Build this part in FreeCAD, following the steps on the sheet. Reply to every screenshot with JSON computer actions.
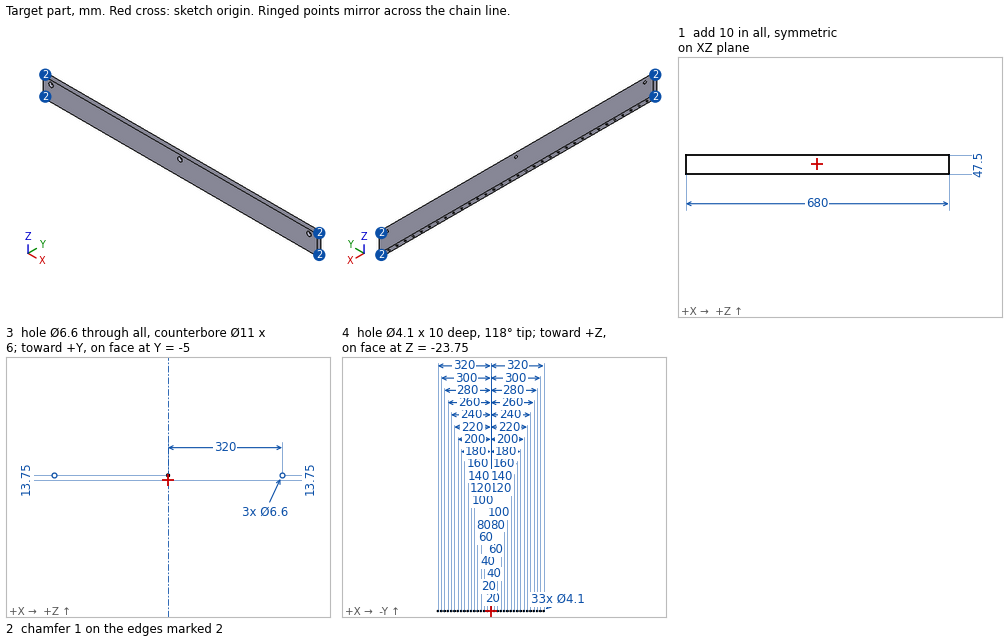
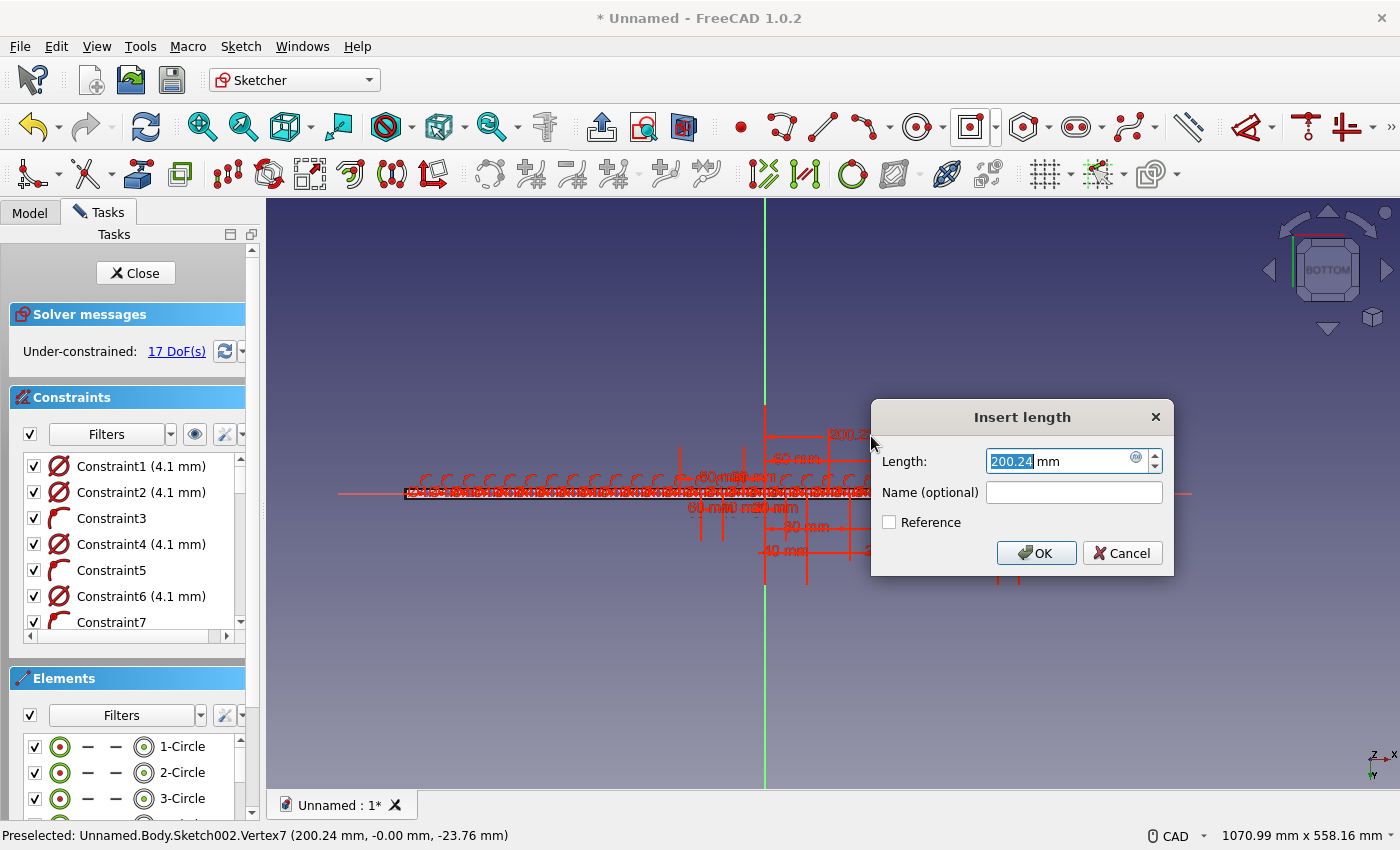
{"action": "type", "text": "200"}
{"action": "key", "text": "Return"}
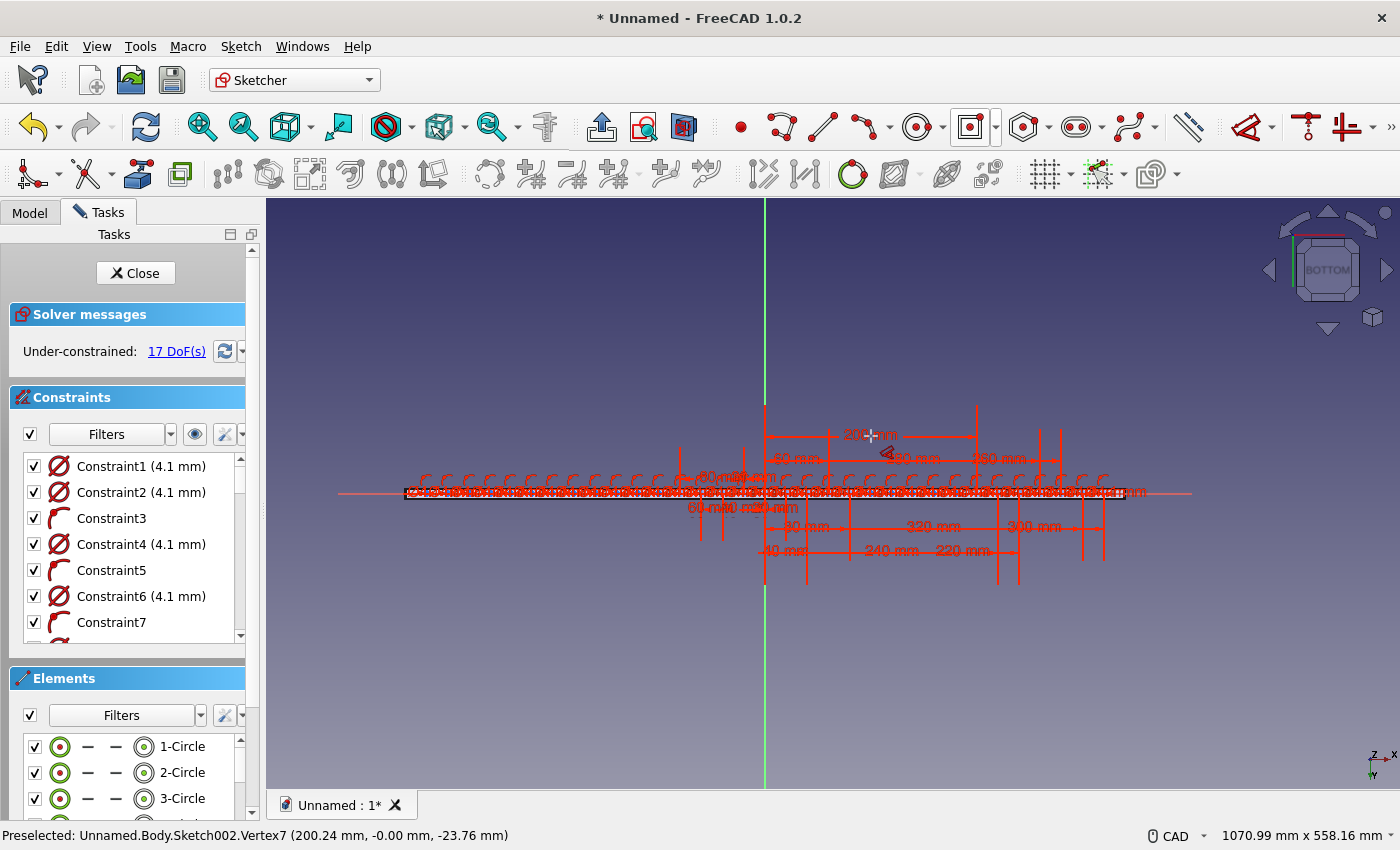
{"action": "left_click", "coordinate": [956, 494]}
{"action": "left_click", "coordinate": [794, 436]}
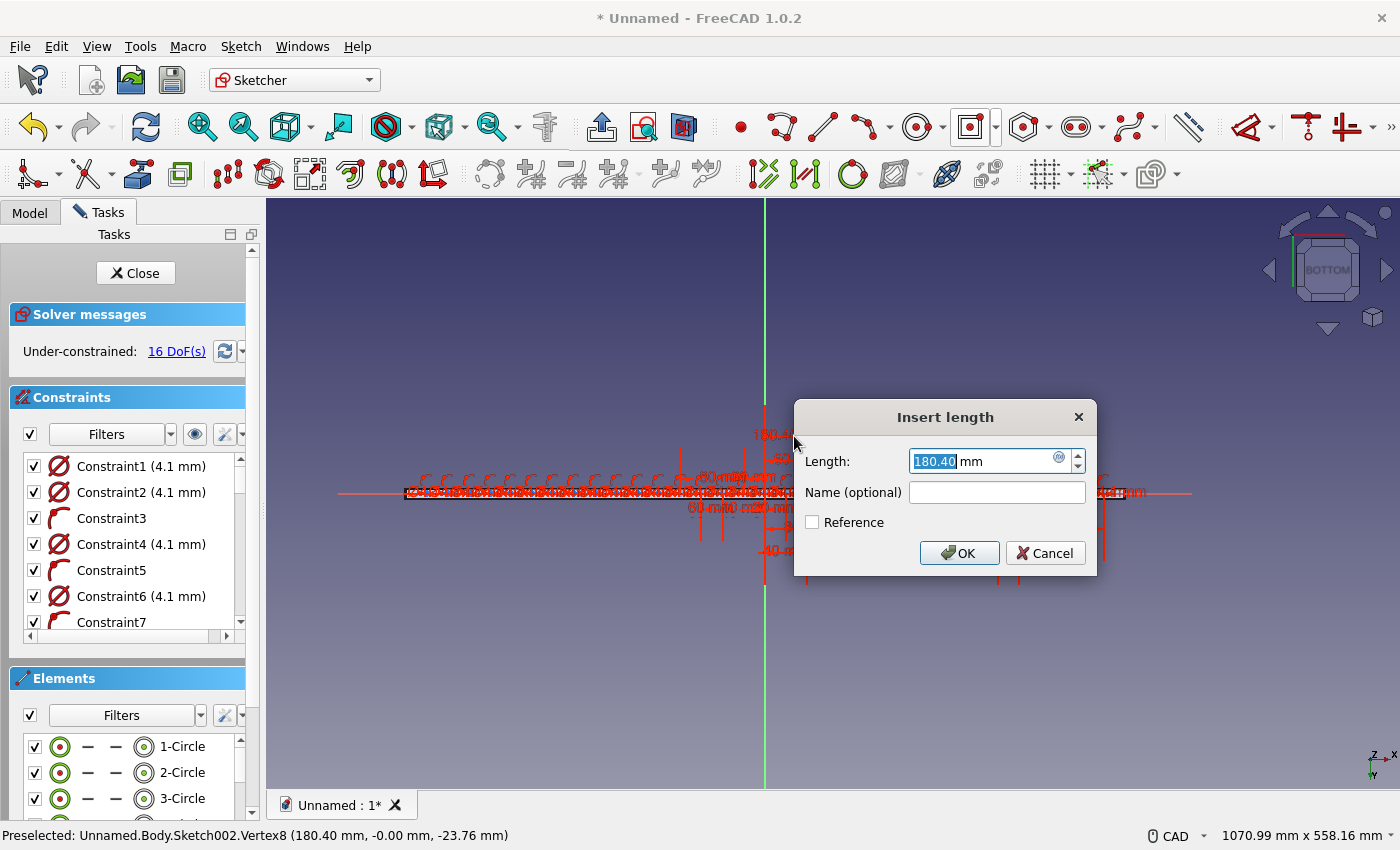
{"action": "type", "text": "180"}
{"action": "key", "text": "Return"}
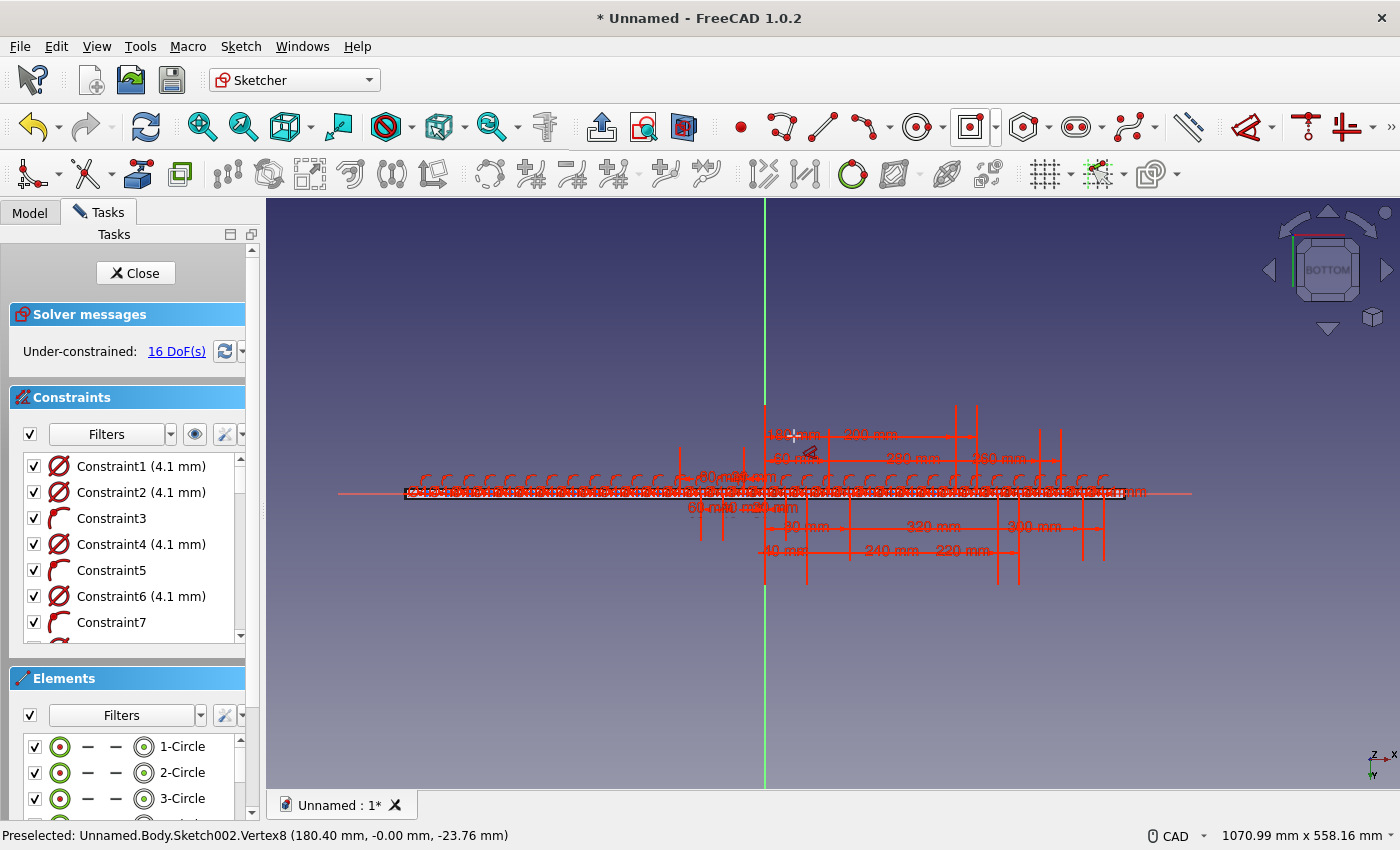
{"action": "left_click", "coordinate": [934, 494]}
{"action": "left_click", "coordinate": [849, 576]}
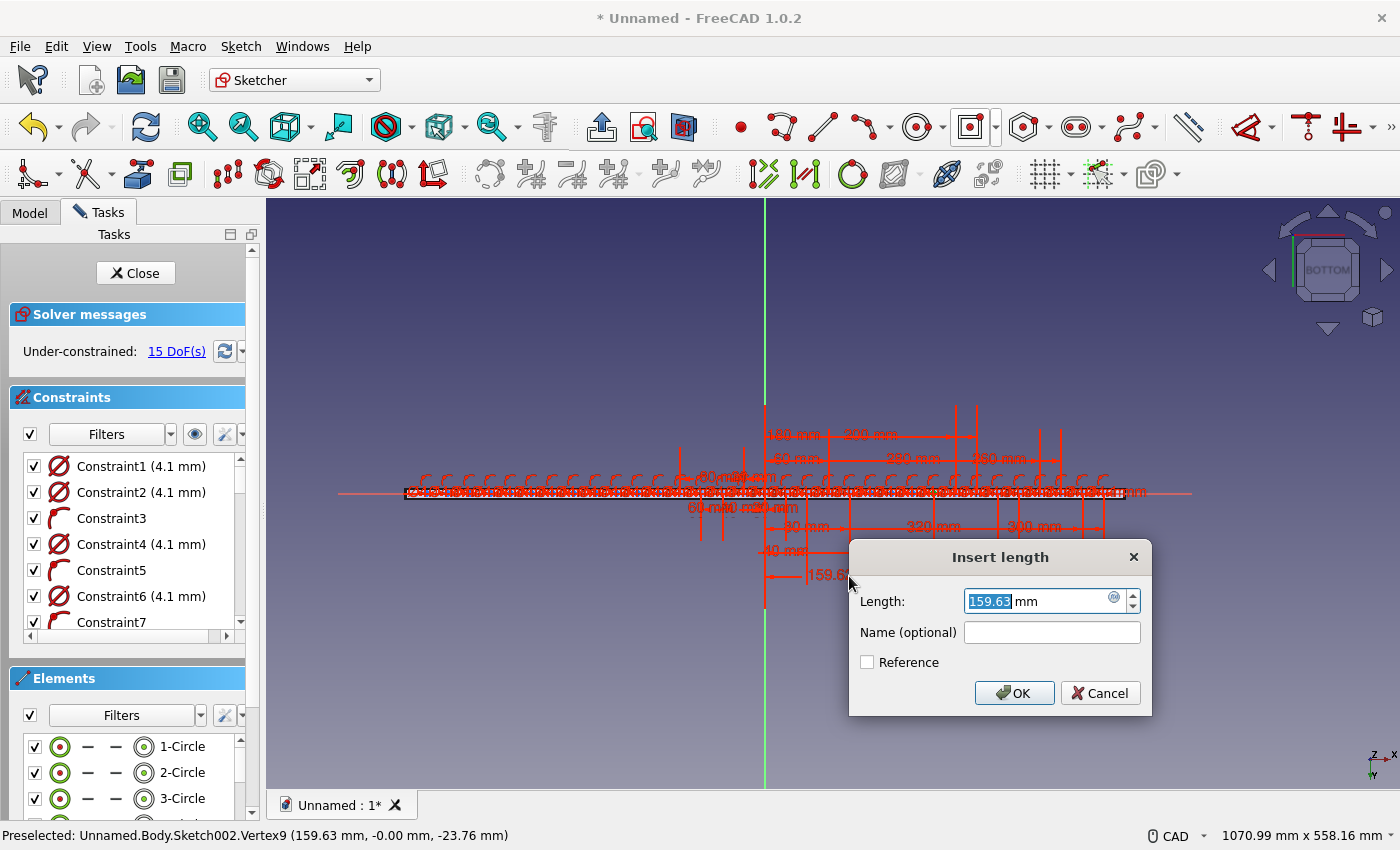
{"action": "type", "text": "160"}
{"action": "key", "text": "Return"}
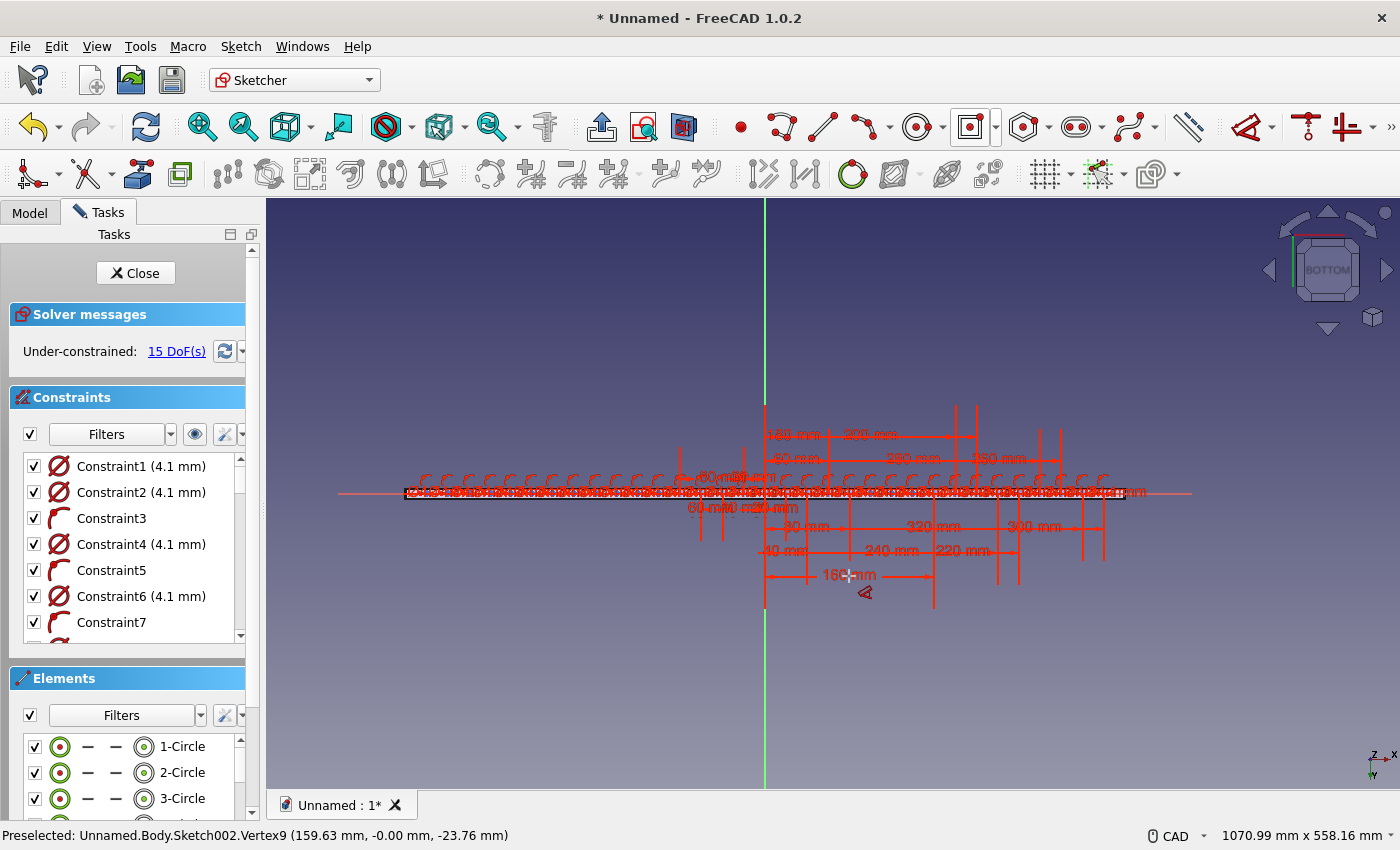
{"action": "left_click", "coordinate": [913, 494]}
{"action": "left_click", "coordinate": [839, 412]}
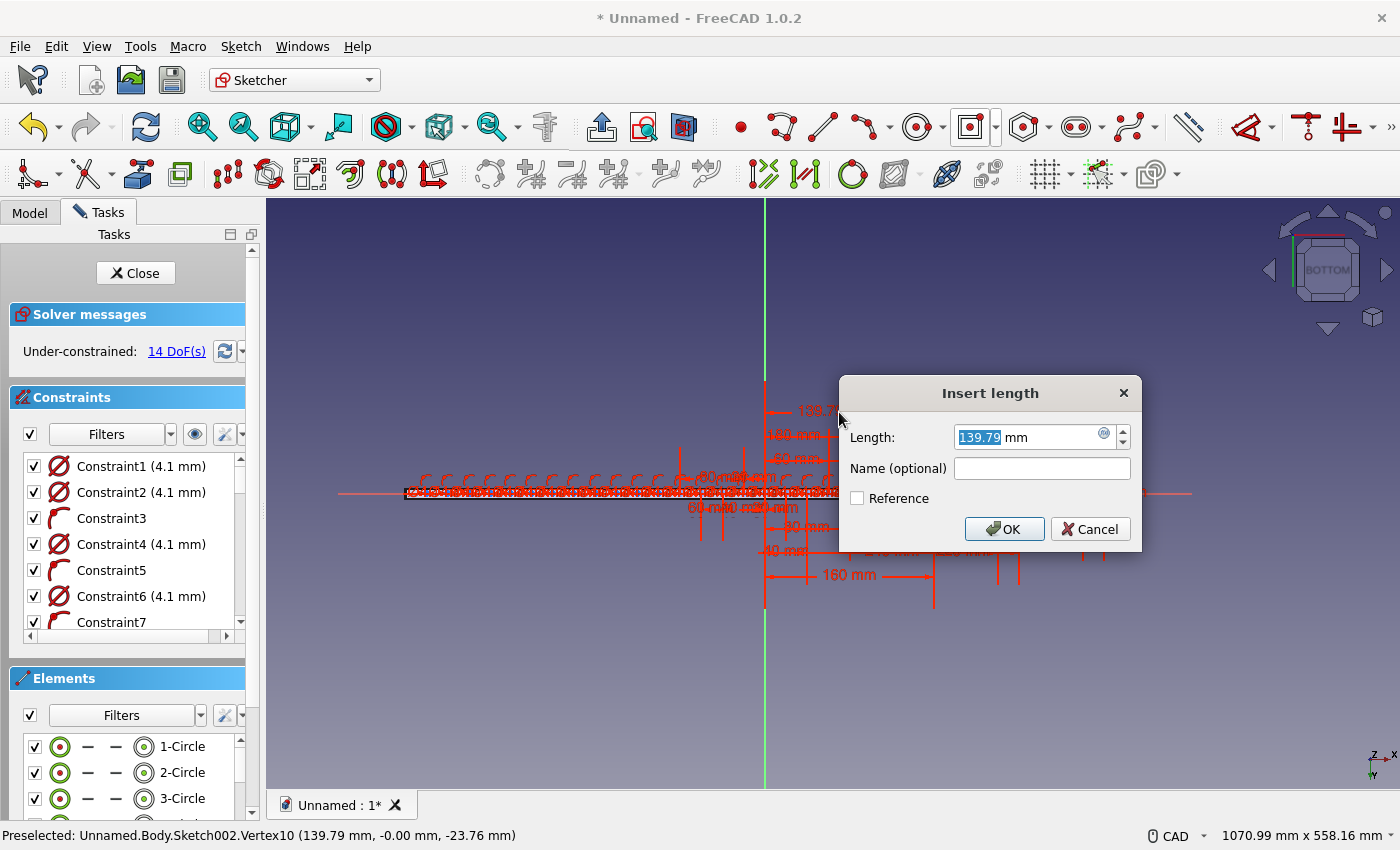
{"action": "type", "text": "140"}
{"action": "key", "text": "Return"}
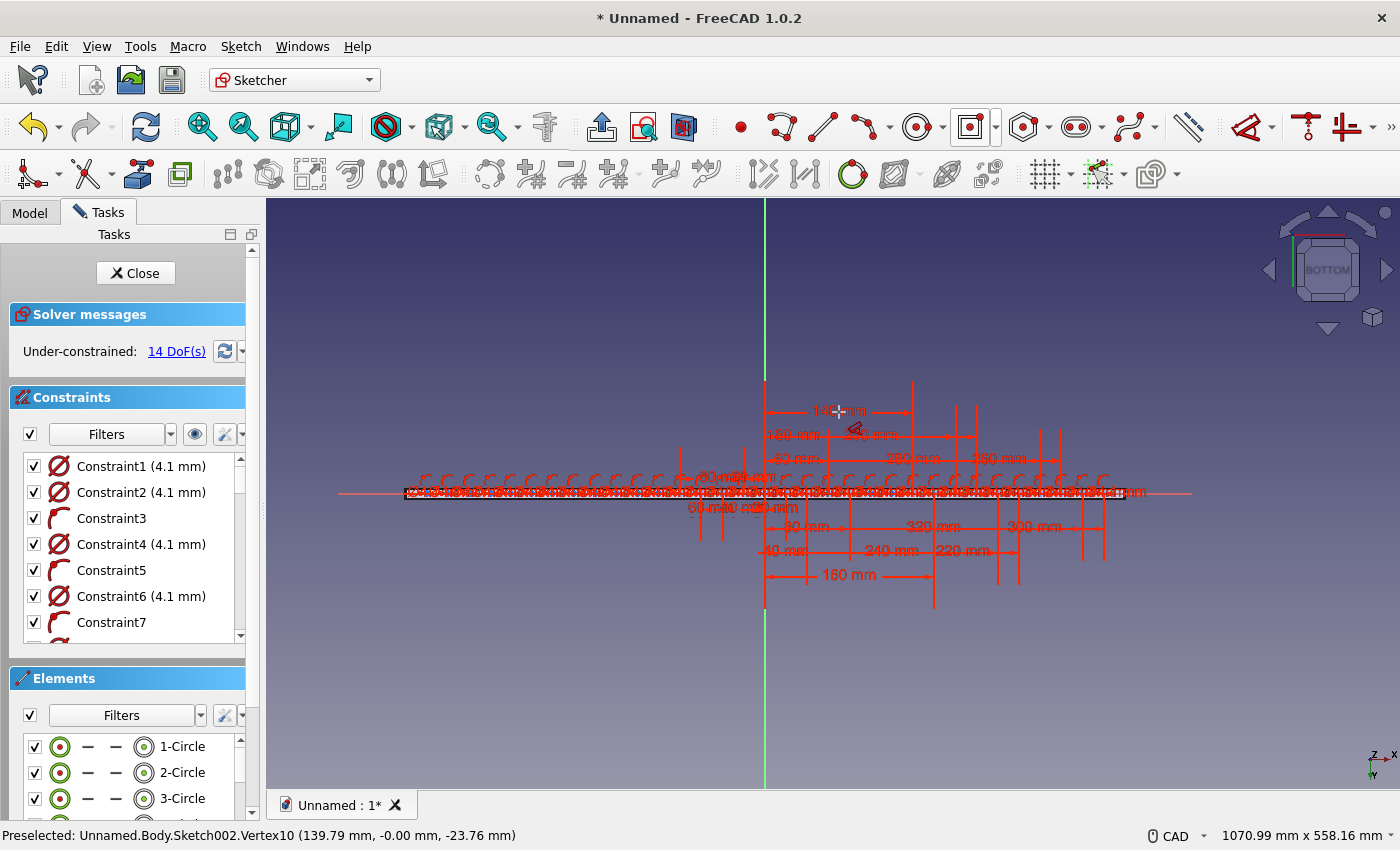
{"action": "left_click", "coordinate": [892, 494]}
{"action": "left_click", "coordinate": [828, 600]}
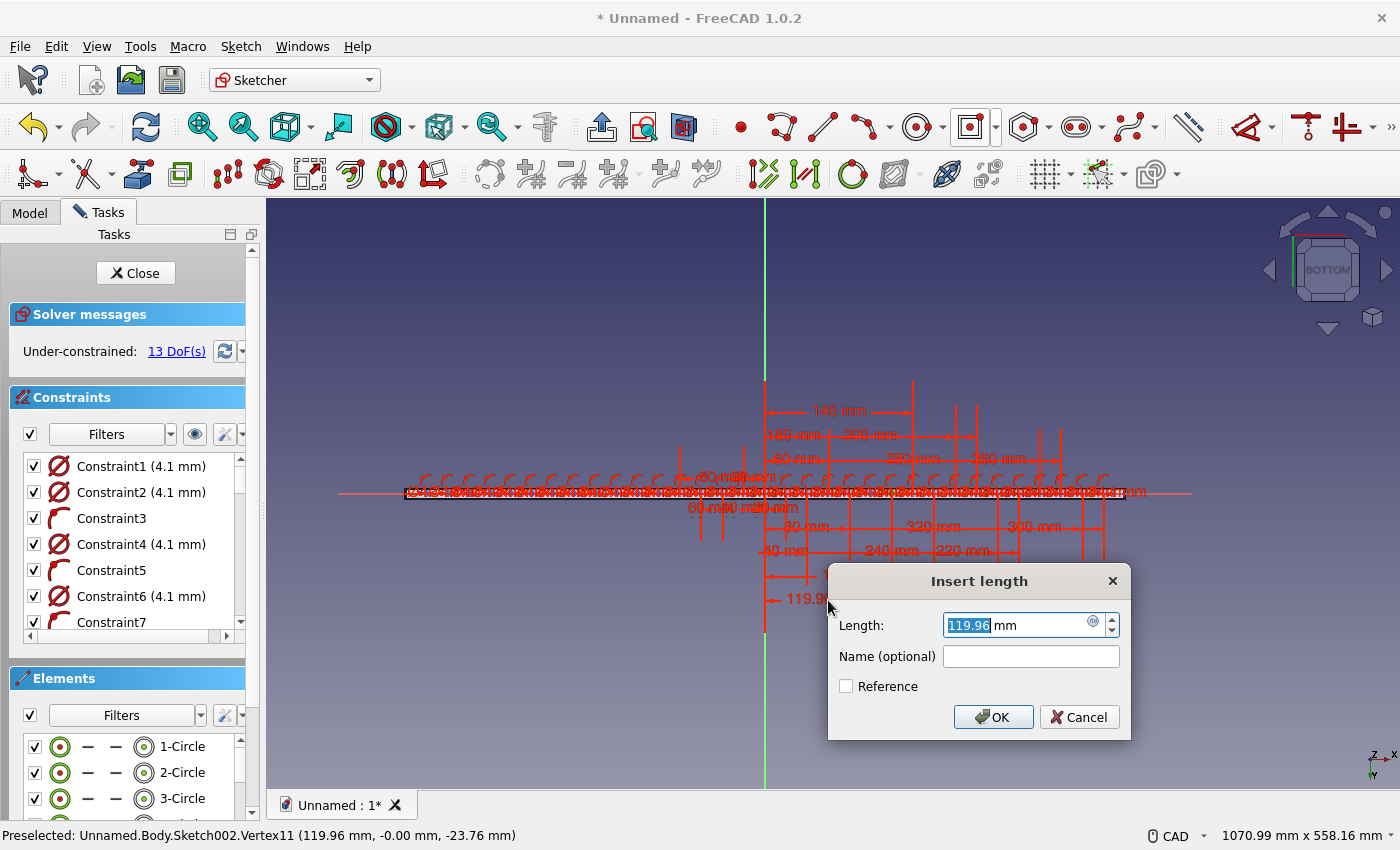
{"action": "type", "text": "120"}
{"action": "key", "text": "Return"}